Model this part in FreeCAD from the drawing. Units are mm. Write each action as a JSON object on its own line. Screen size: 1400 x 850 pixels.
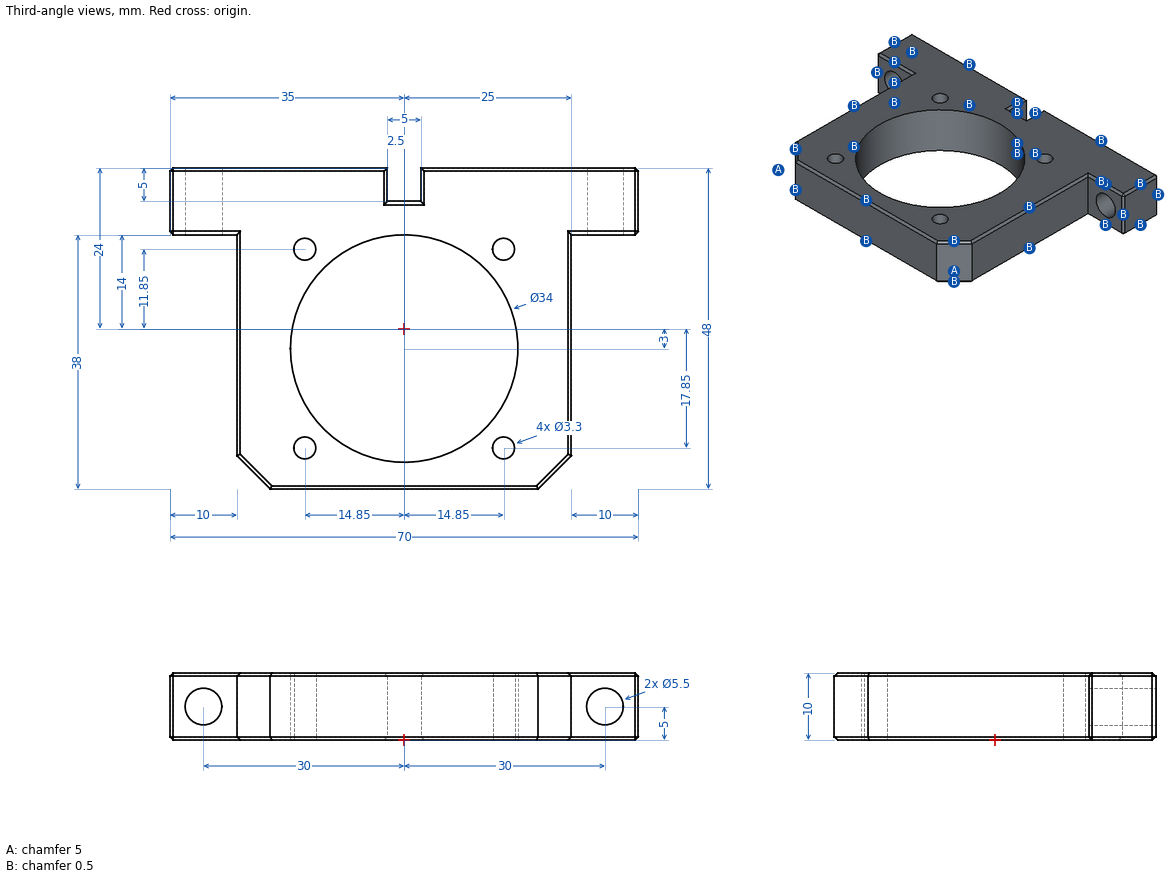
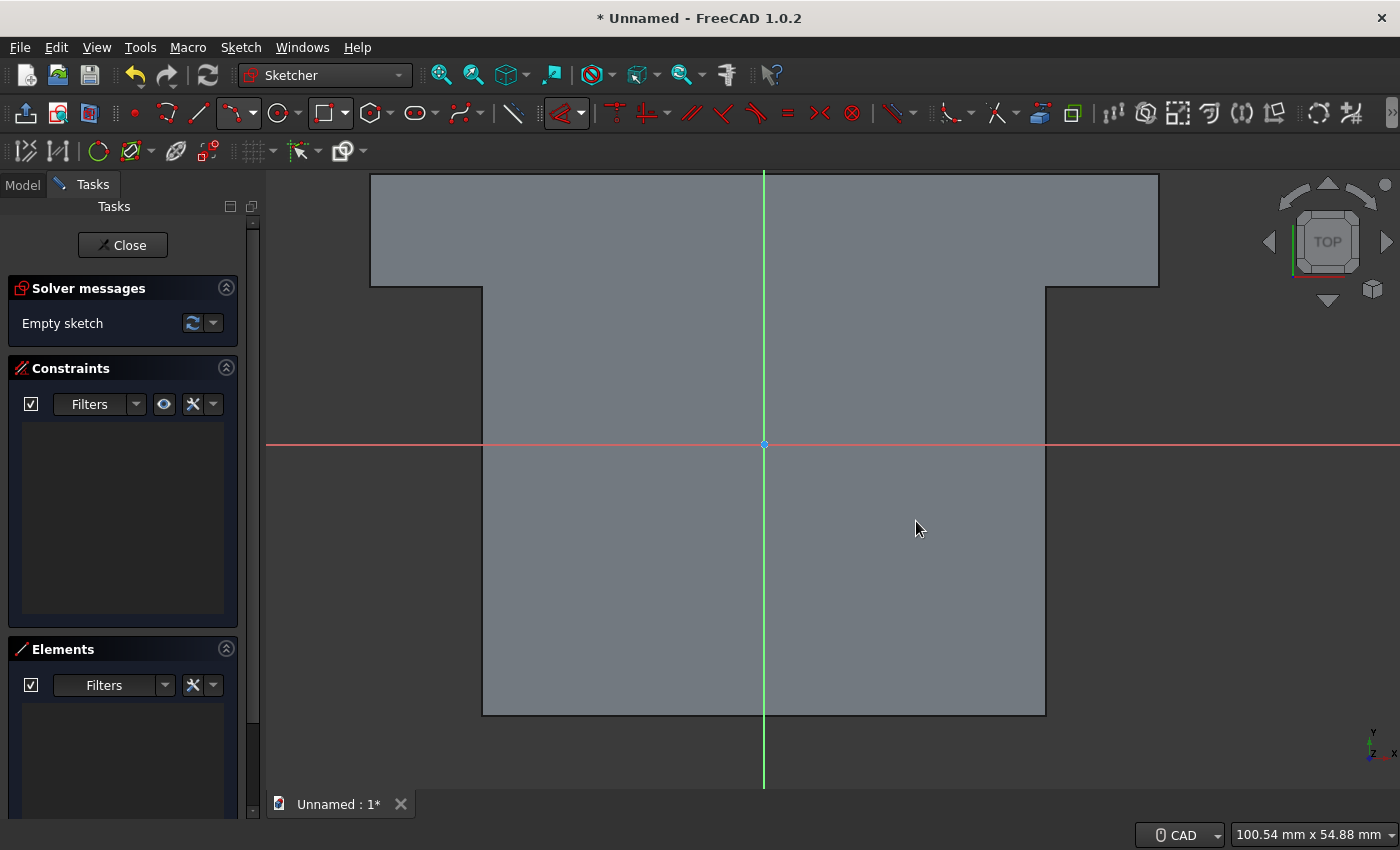
{"action": "left_click", "coordinate": [278, 114]}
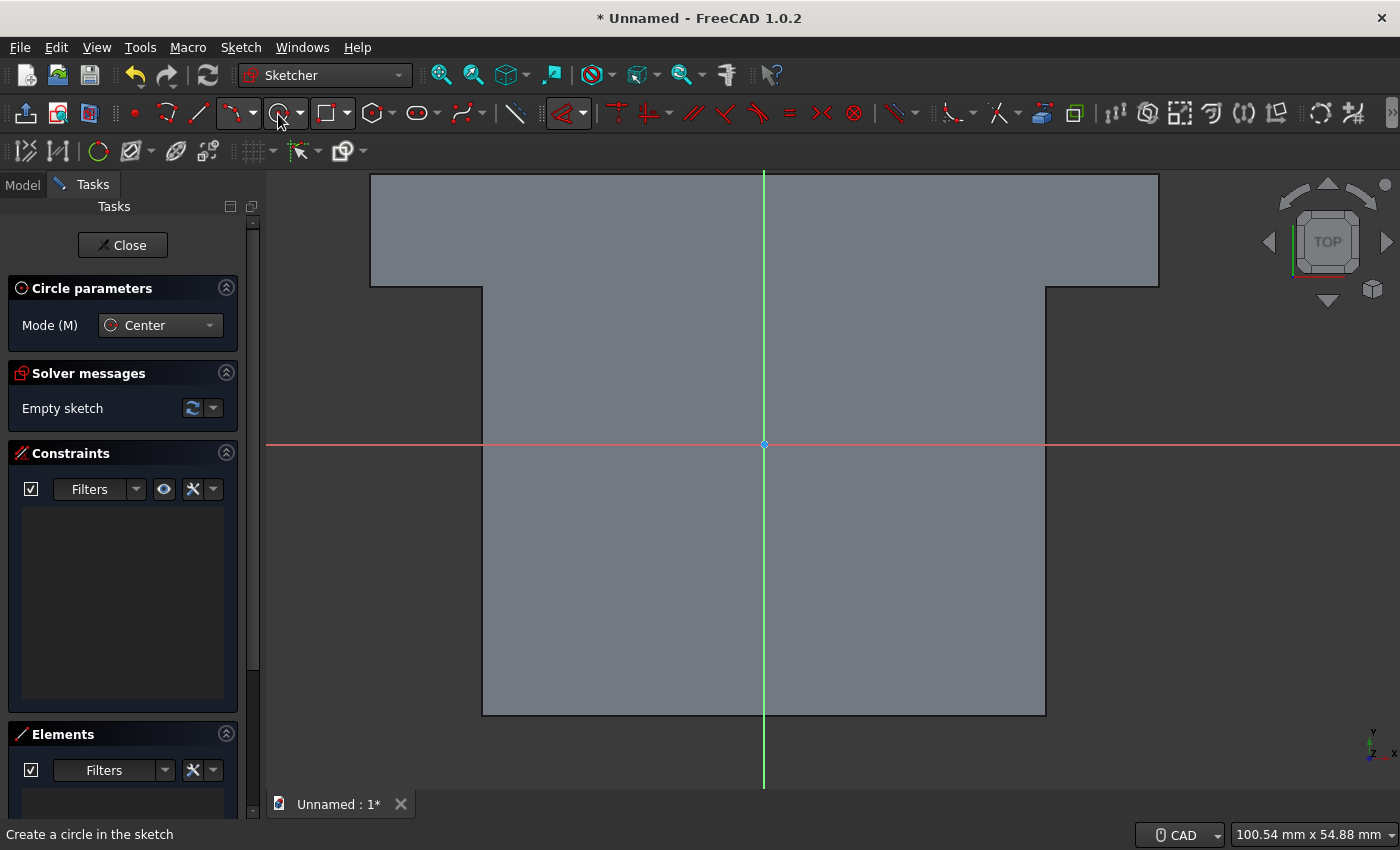
{"action": "left_click", "coordinate": [764, 479]}
{"action": "left_click", "coordinate": [900, 343]}
{"action": "key", "text": "Escape"}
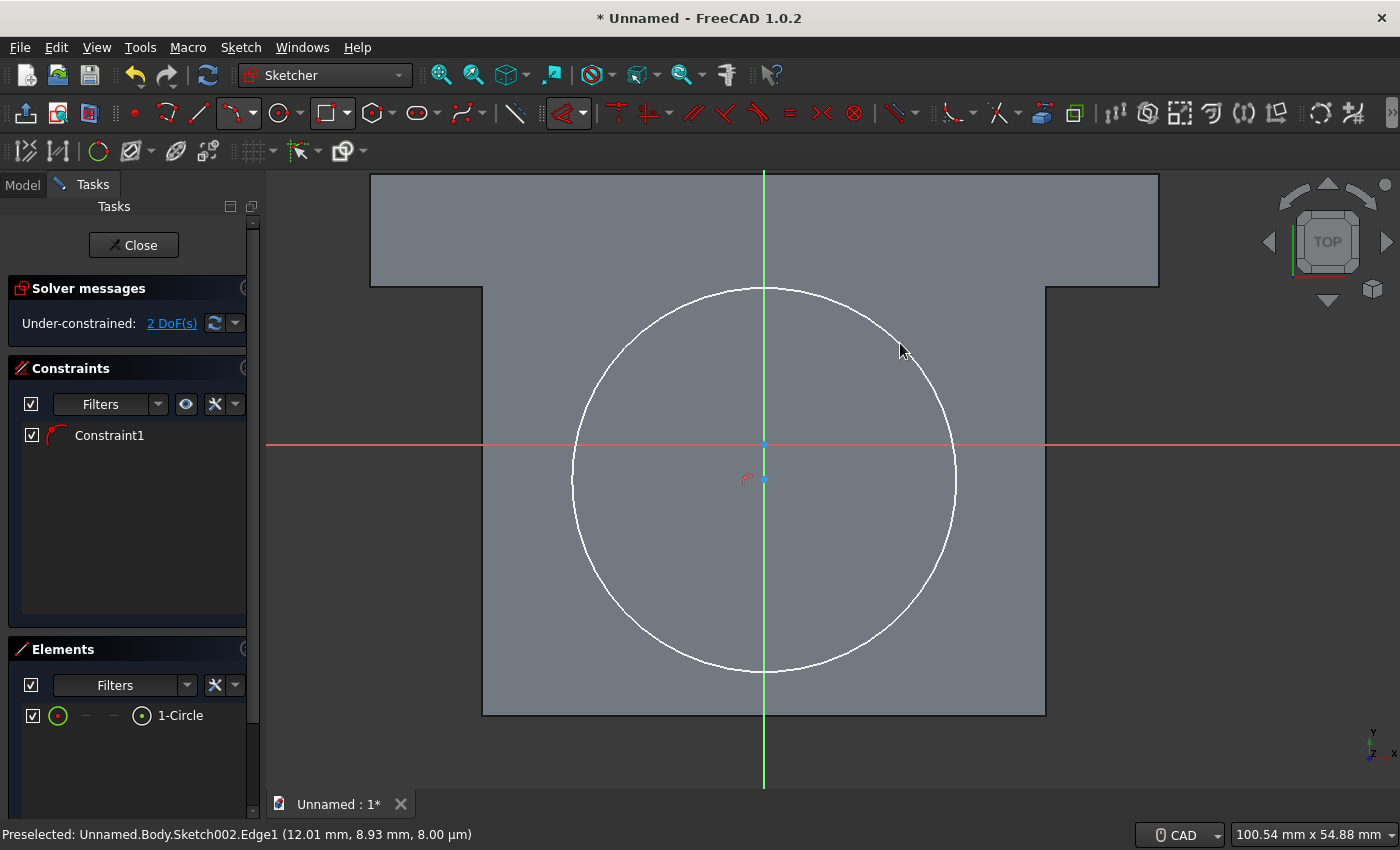
{"action": "left_click", "coordinate": [900, 344]}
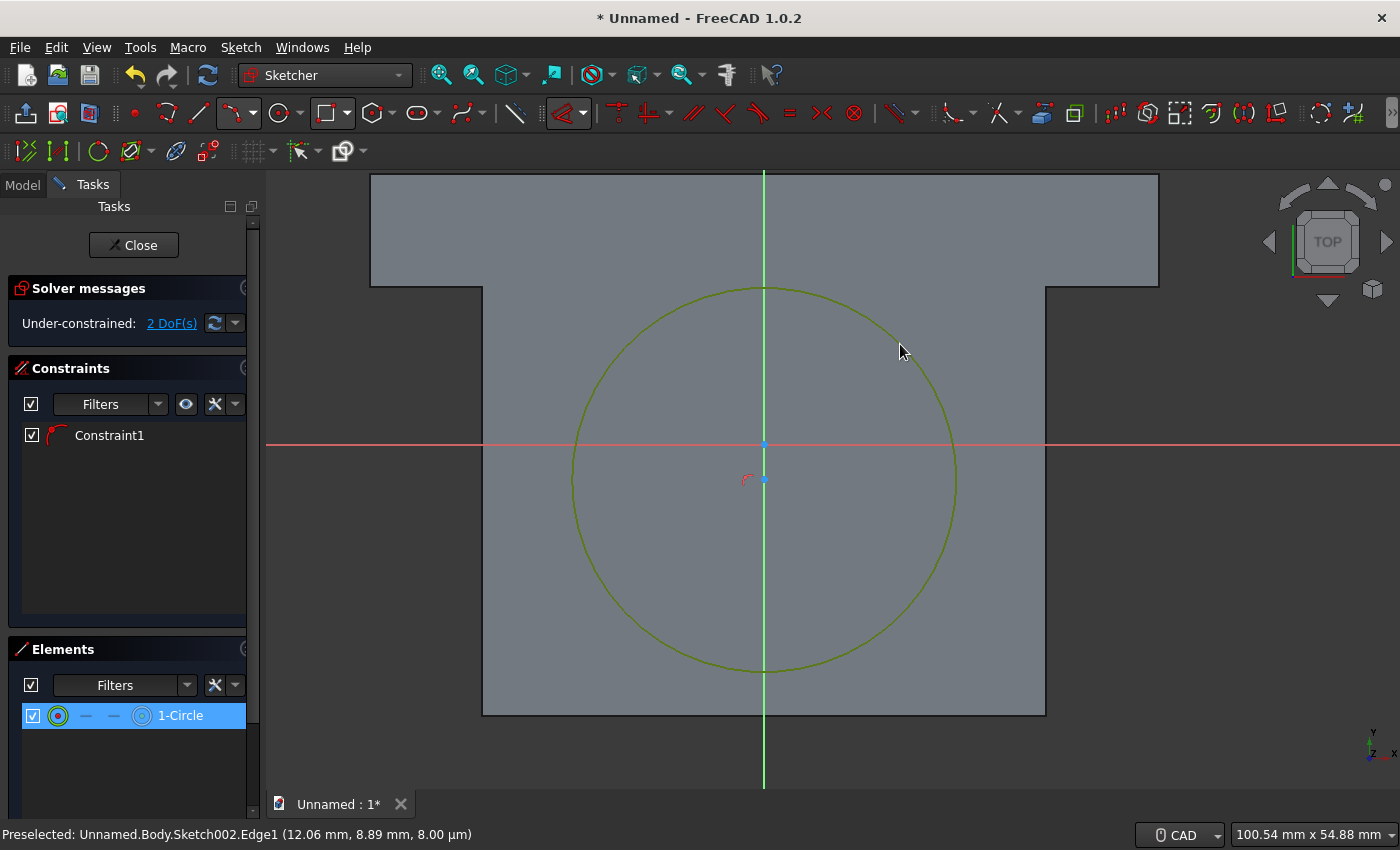
{"action": "left_click", "coordinate": [586, 114]}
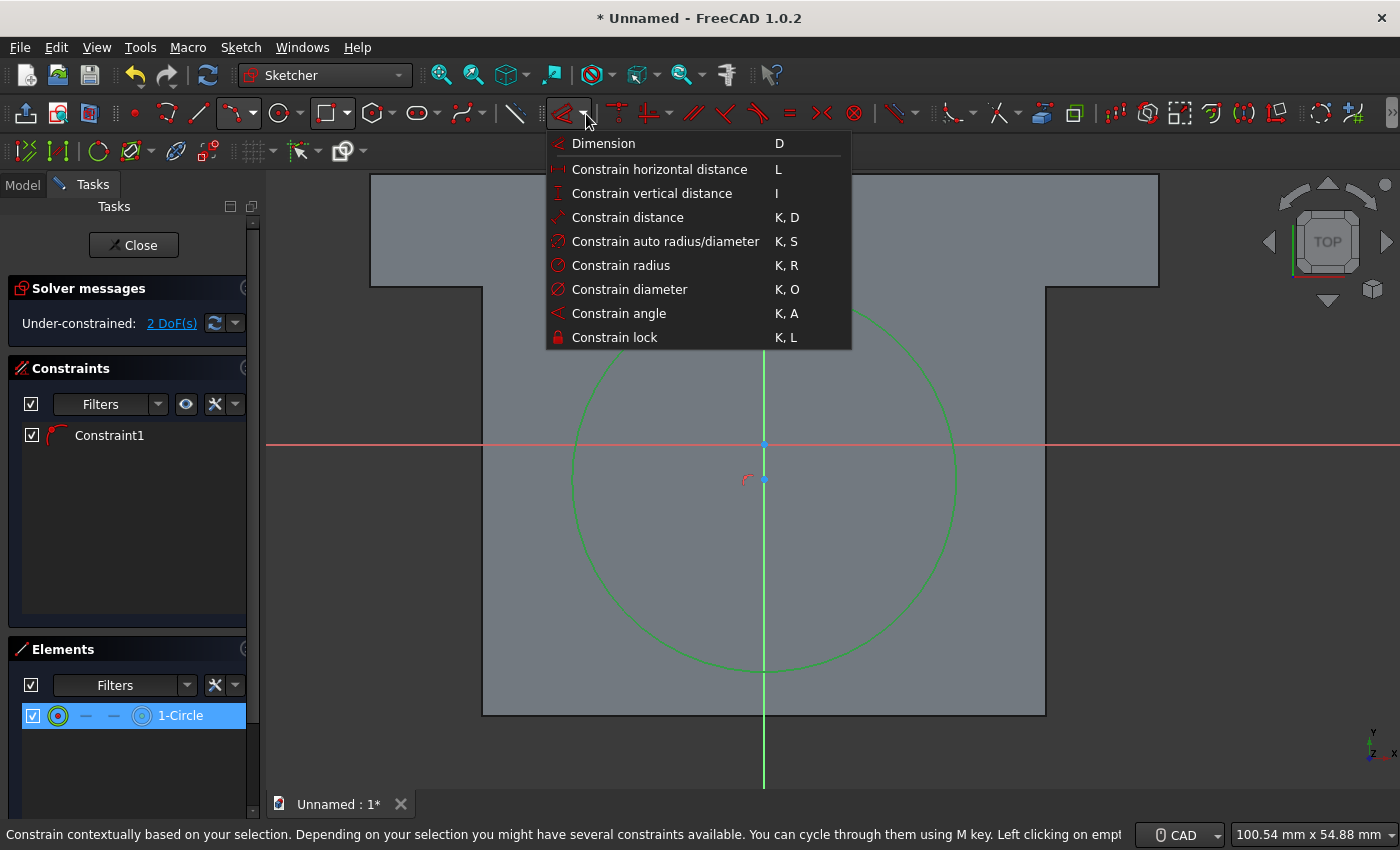
{"action": "left_click", "coordinate": [699, 289]}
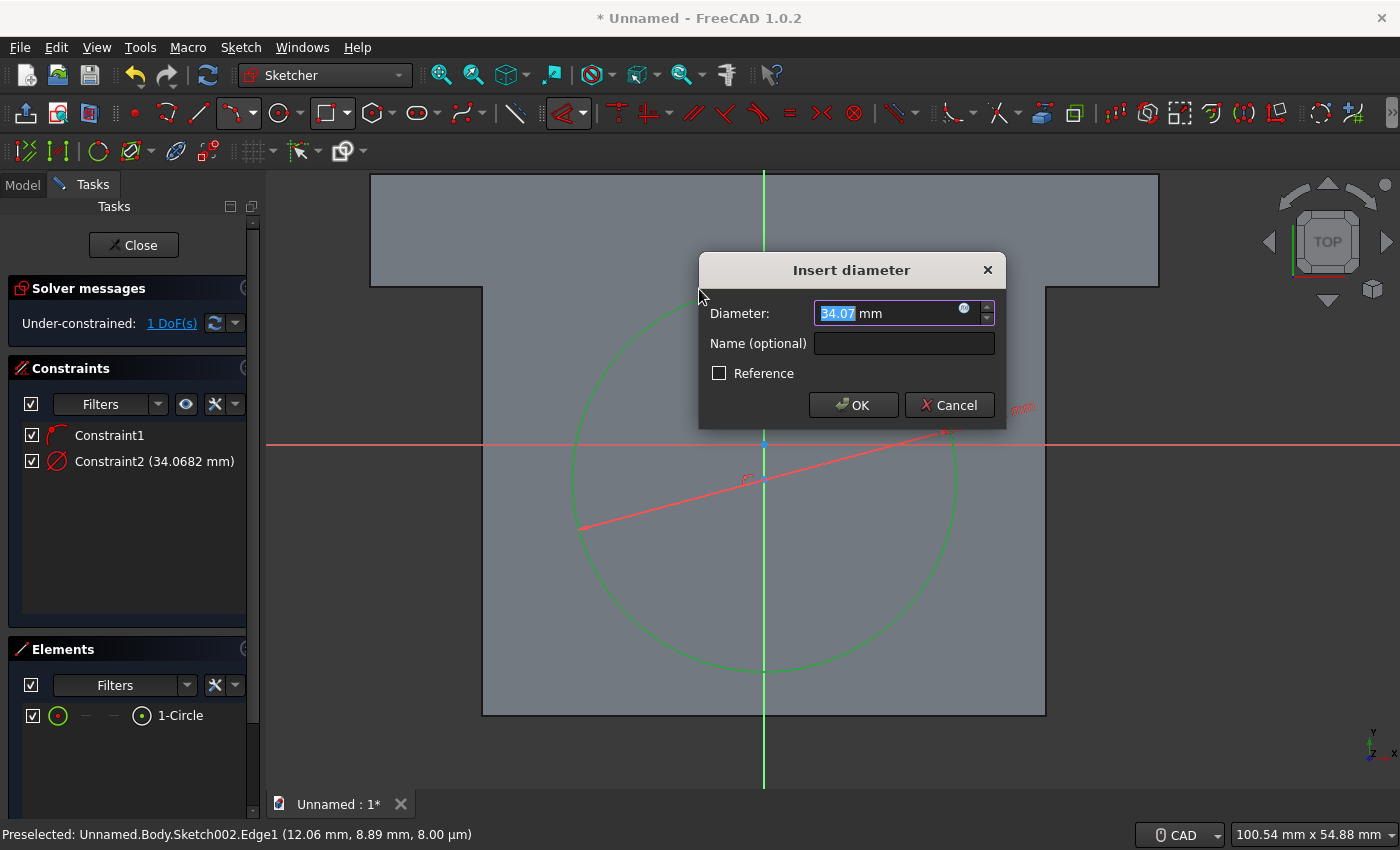
{"action": "type", "text": "34"}
{"action": "key", "text": "Return"}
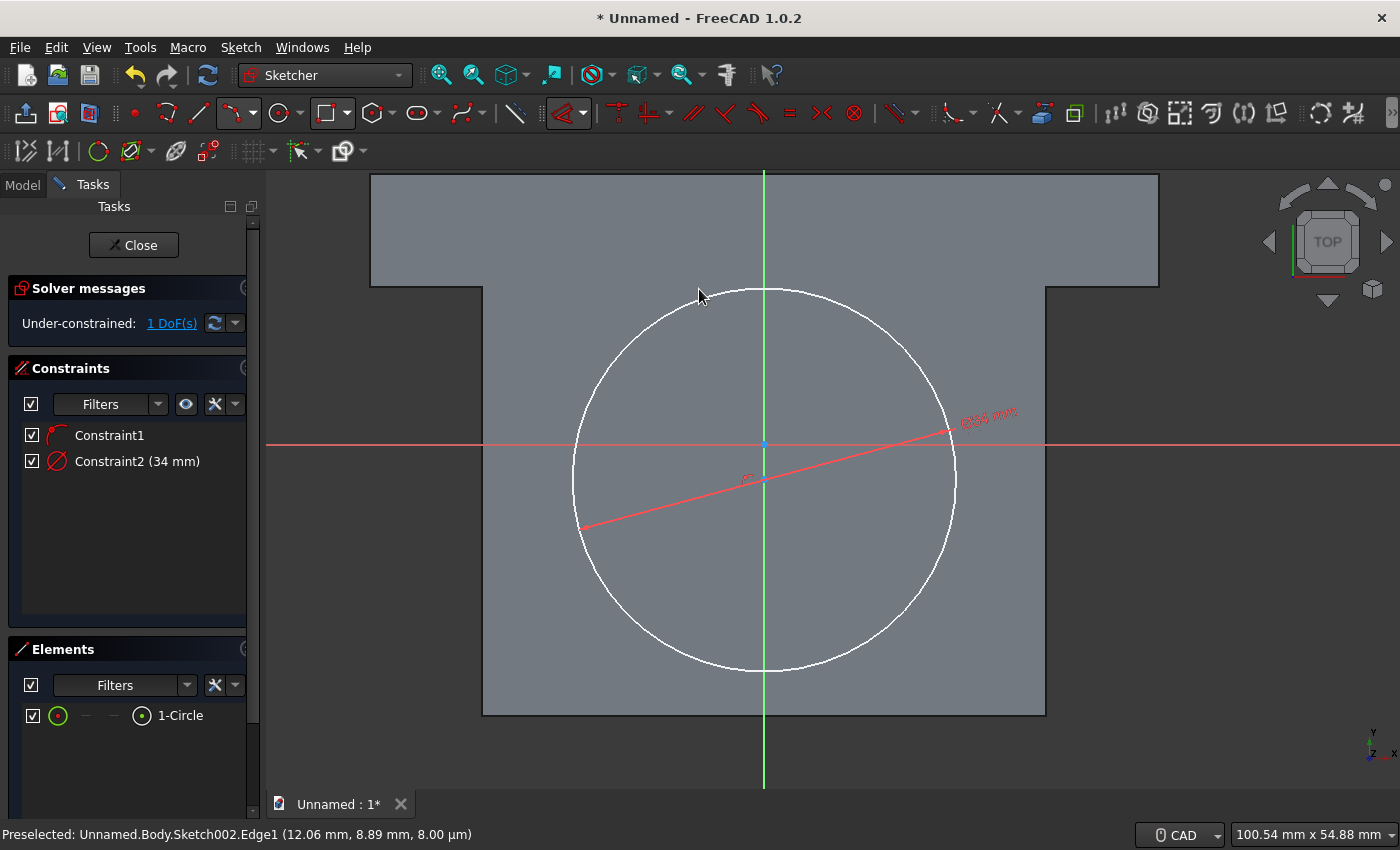
{"action": "left_click", "coordinate": [764, 480]}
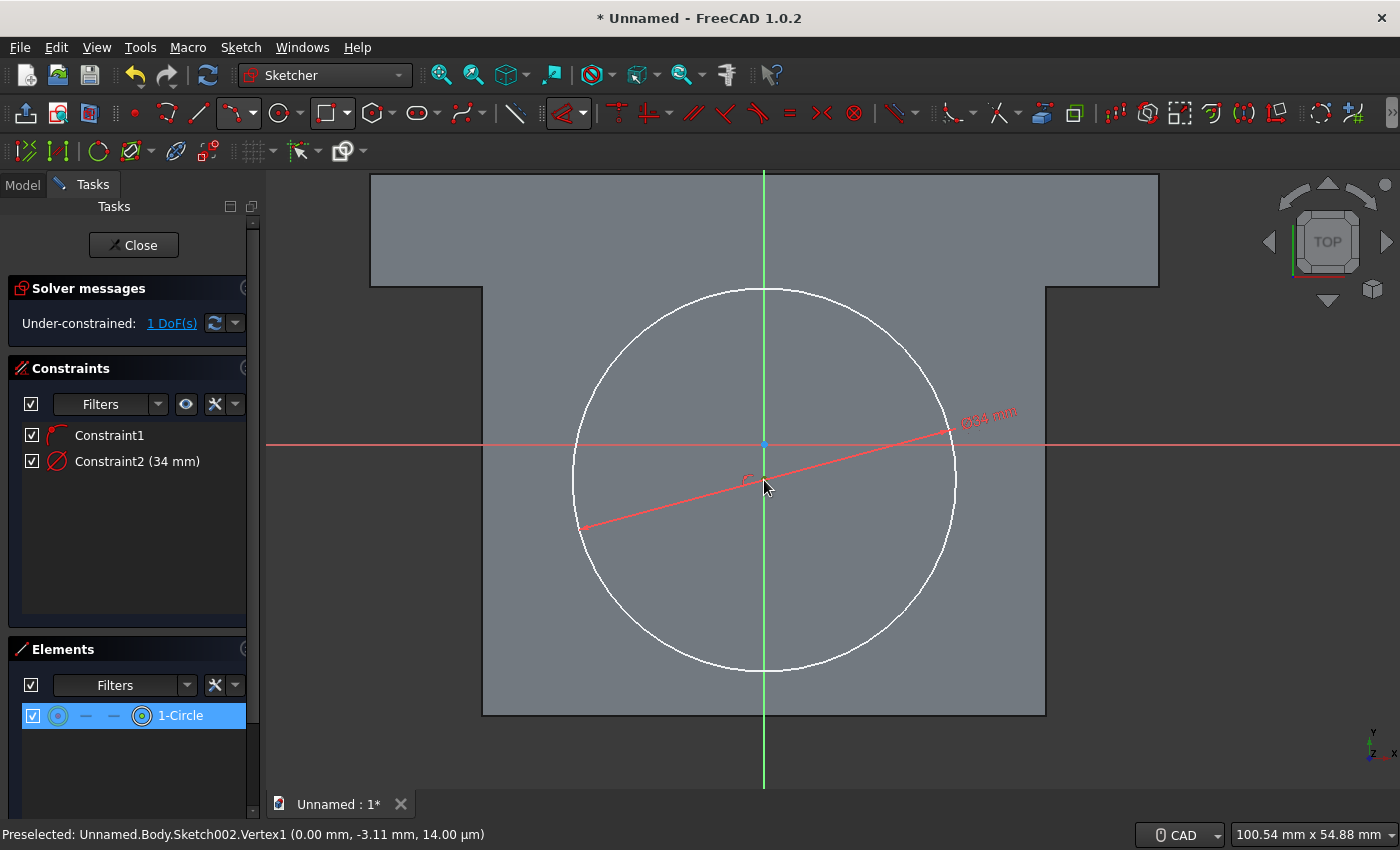
{"action": "left_click", "coordinate": [586, 114]}